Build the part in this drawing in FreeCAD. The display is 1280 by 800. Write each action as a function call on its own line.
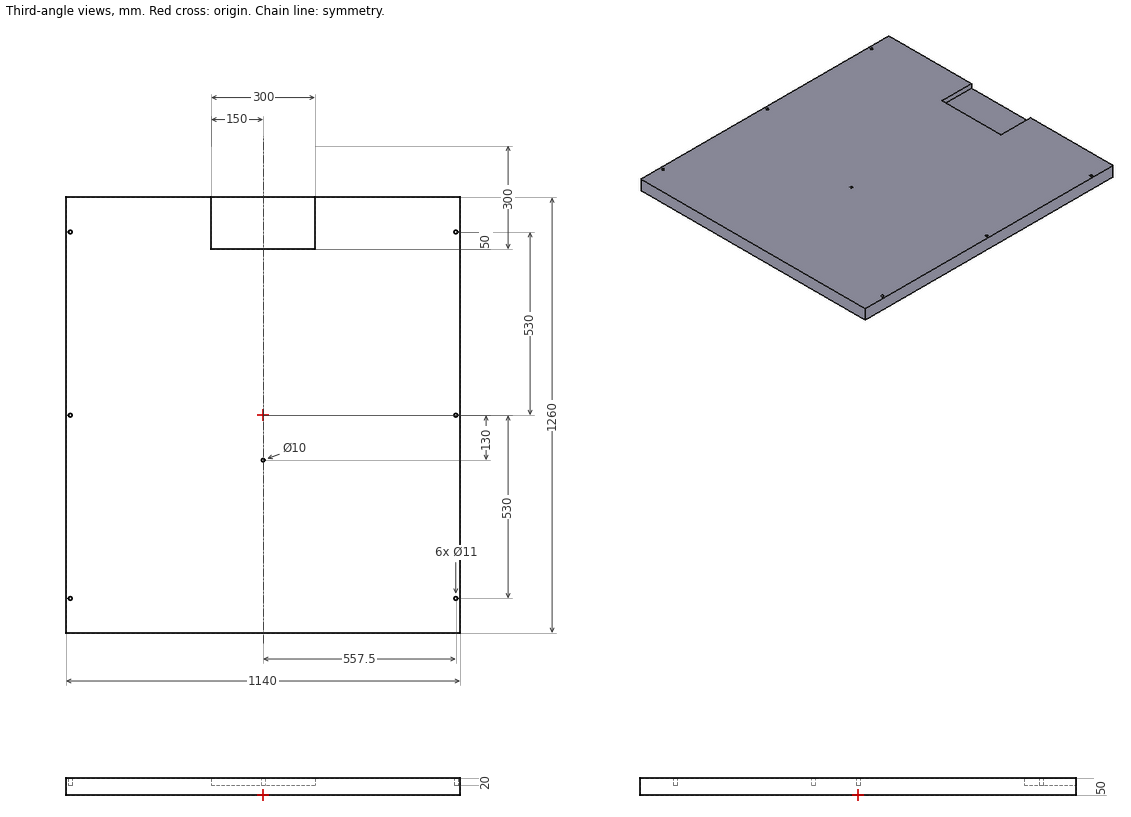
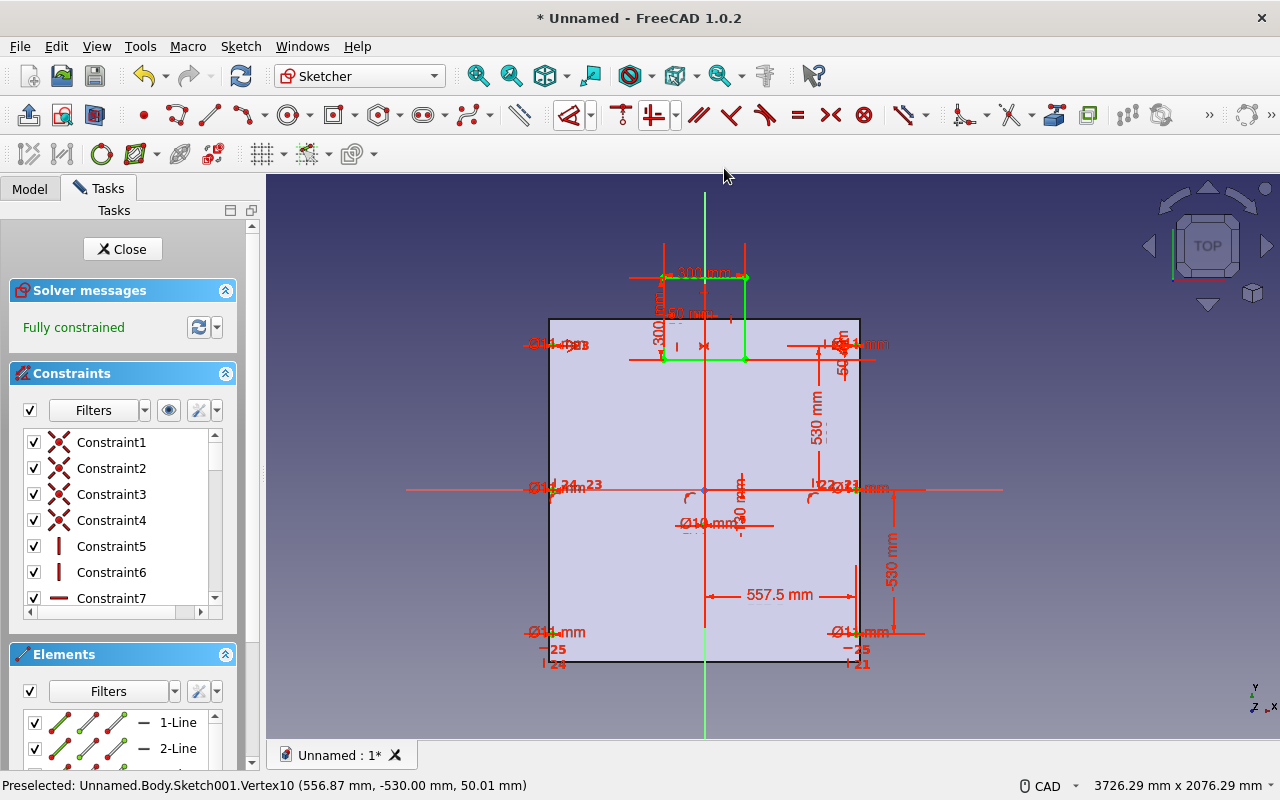
click(123, 249)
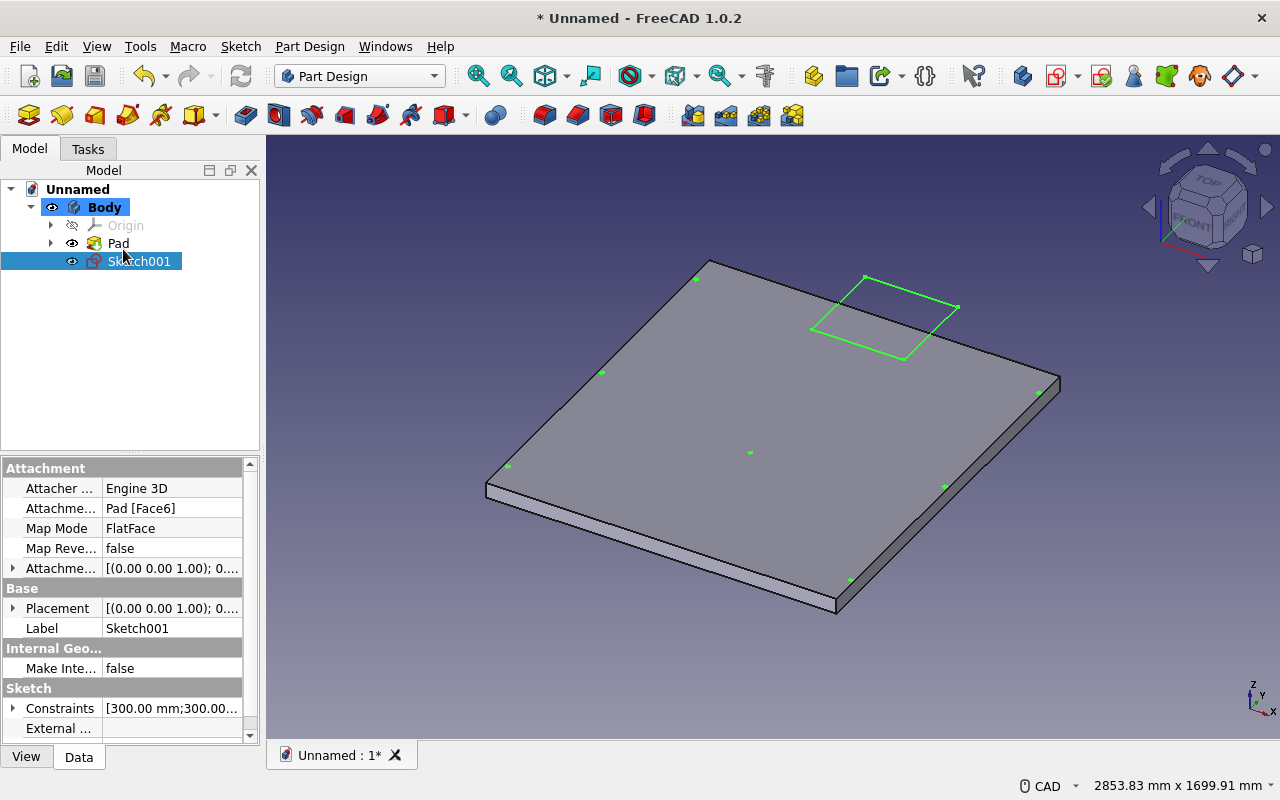
click(246, 116)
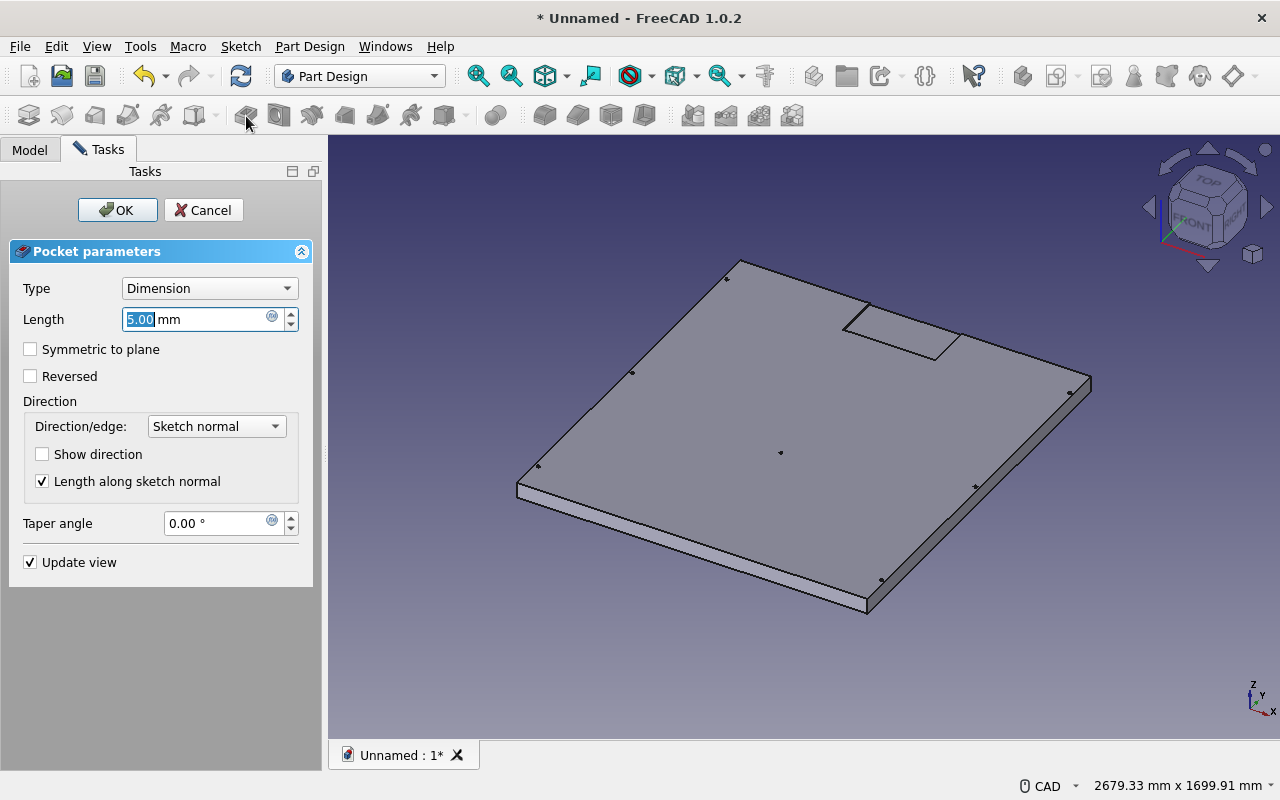
text(20)
key(Tab)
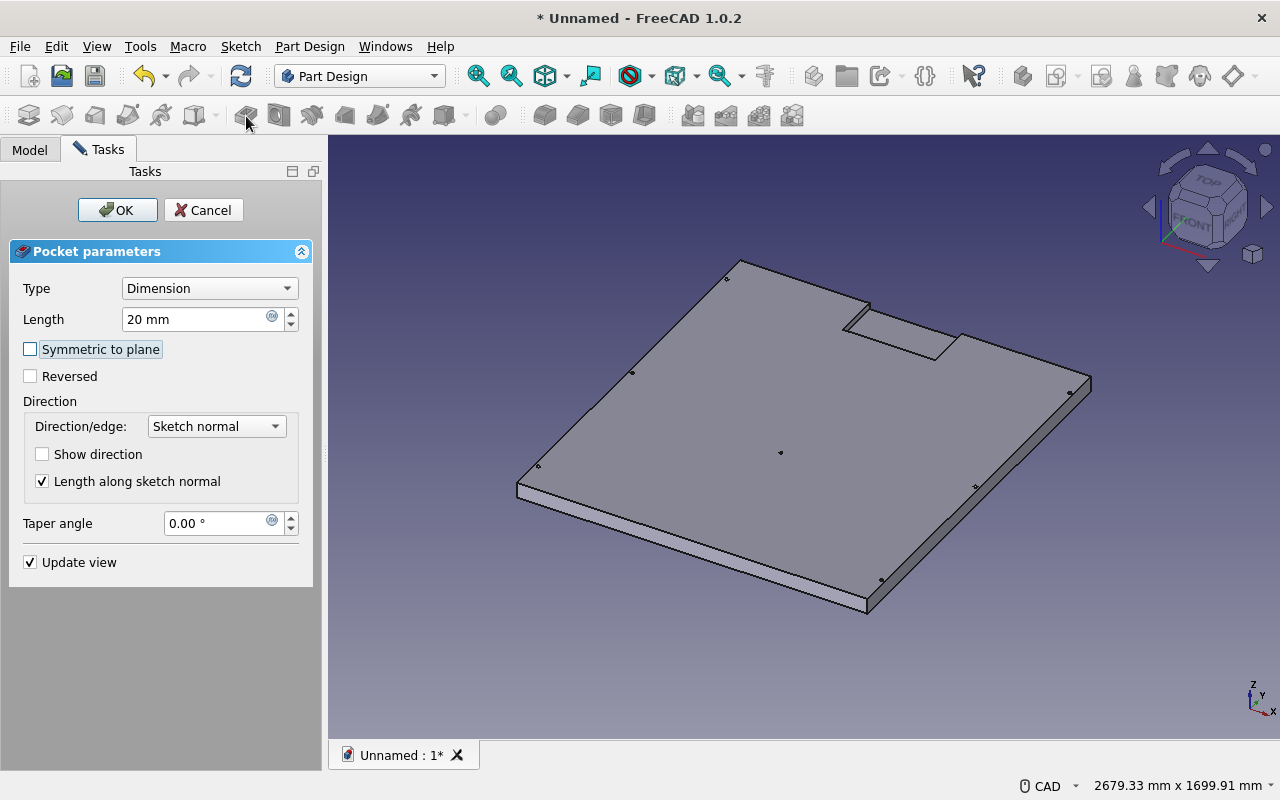
click(118, 210)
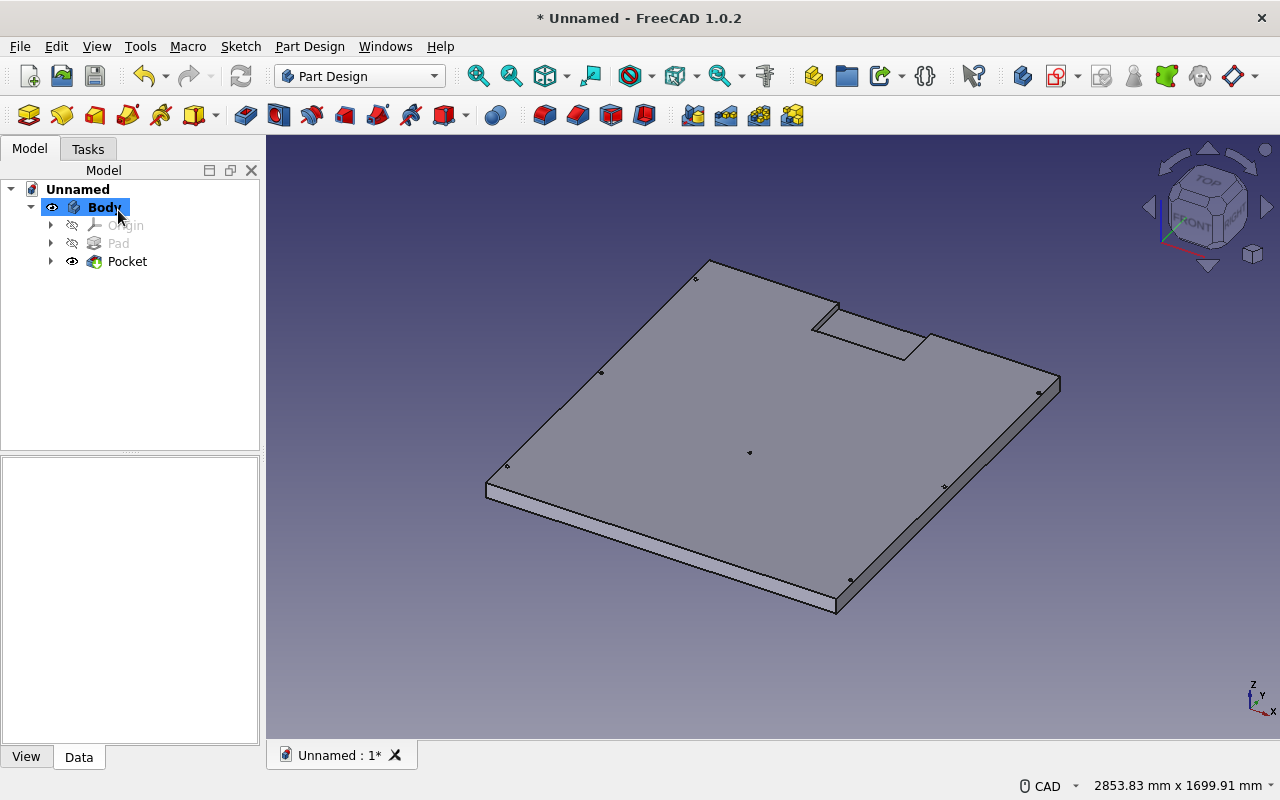
key(0)